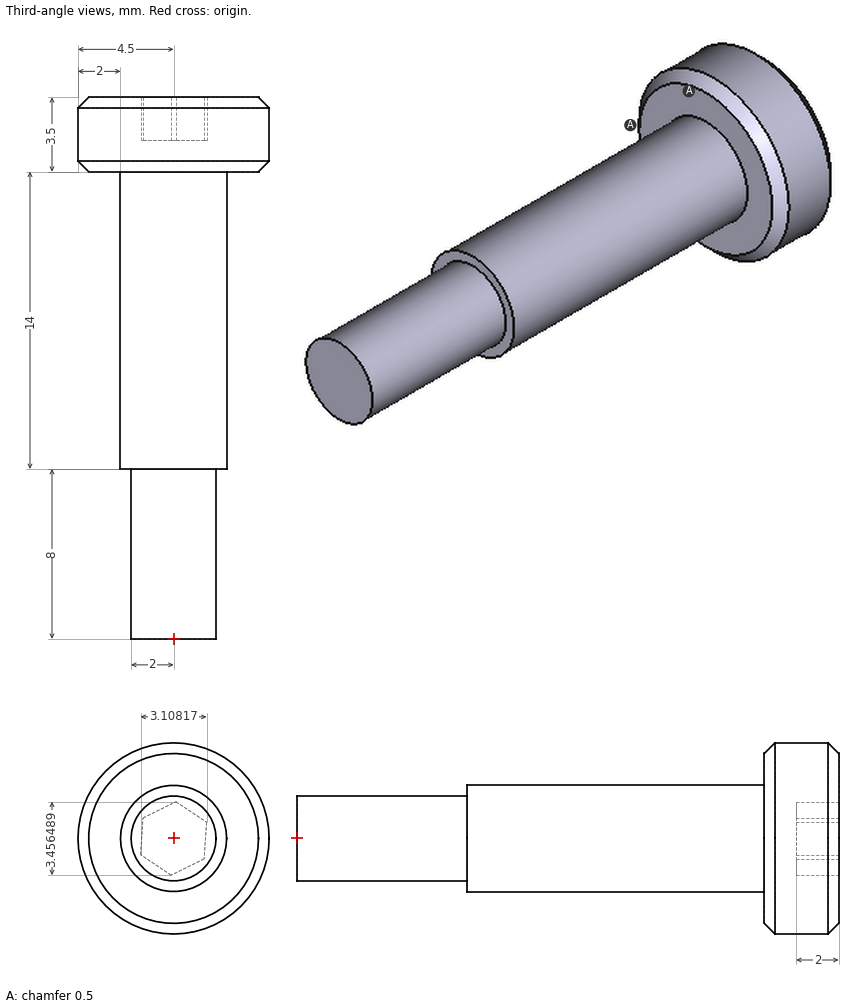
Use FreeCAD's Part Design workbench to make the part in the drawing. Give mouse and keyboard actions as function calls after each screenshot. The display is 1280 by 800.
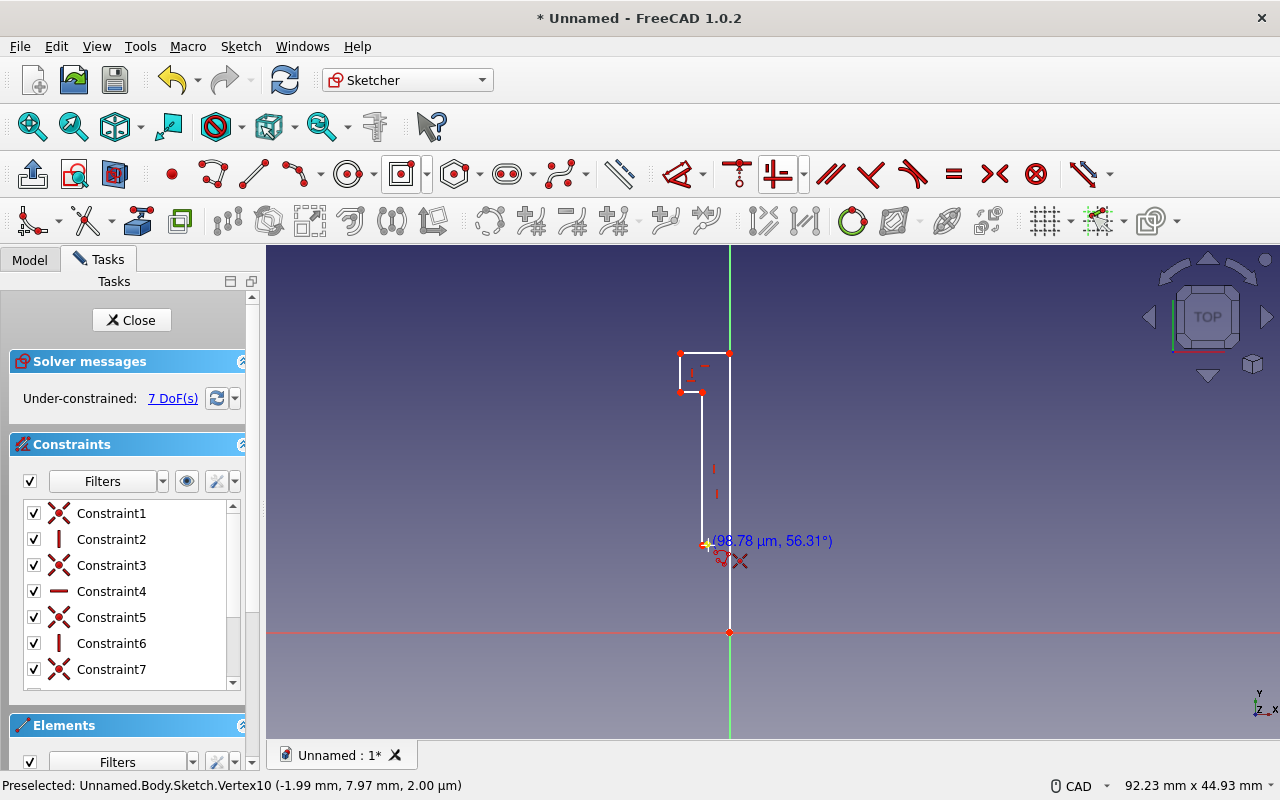
click(708, 624)
click(730, 633)
key(Escape)
key(Escape)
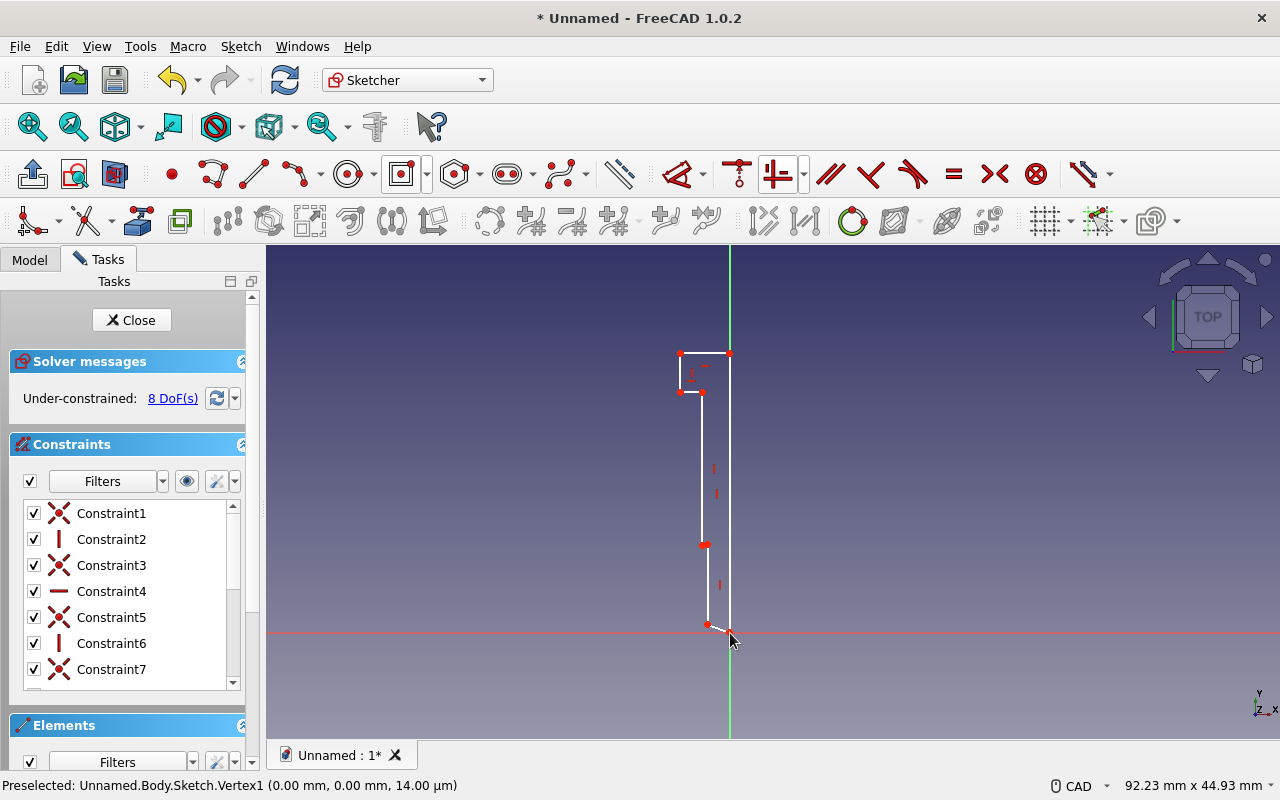
scroll(705, 545, up, 9)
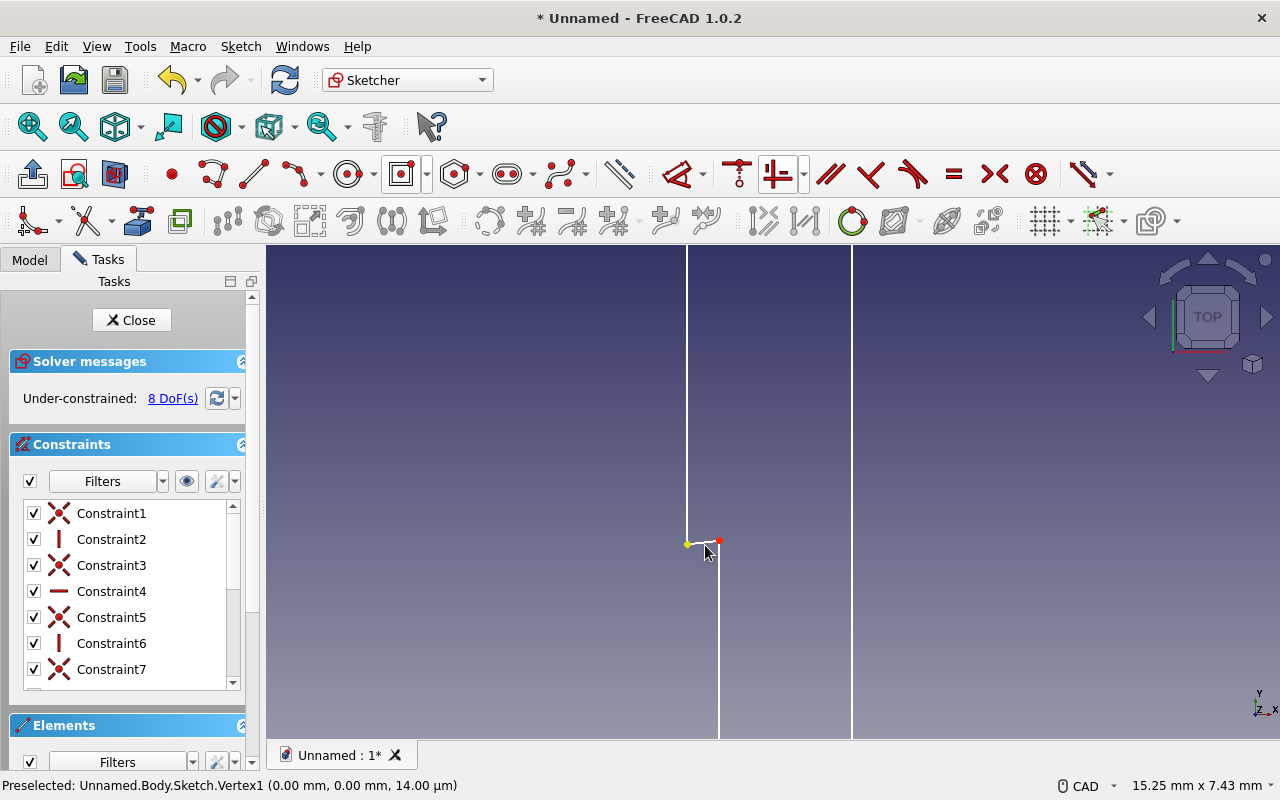
click(703, 543)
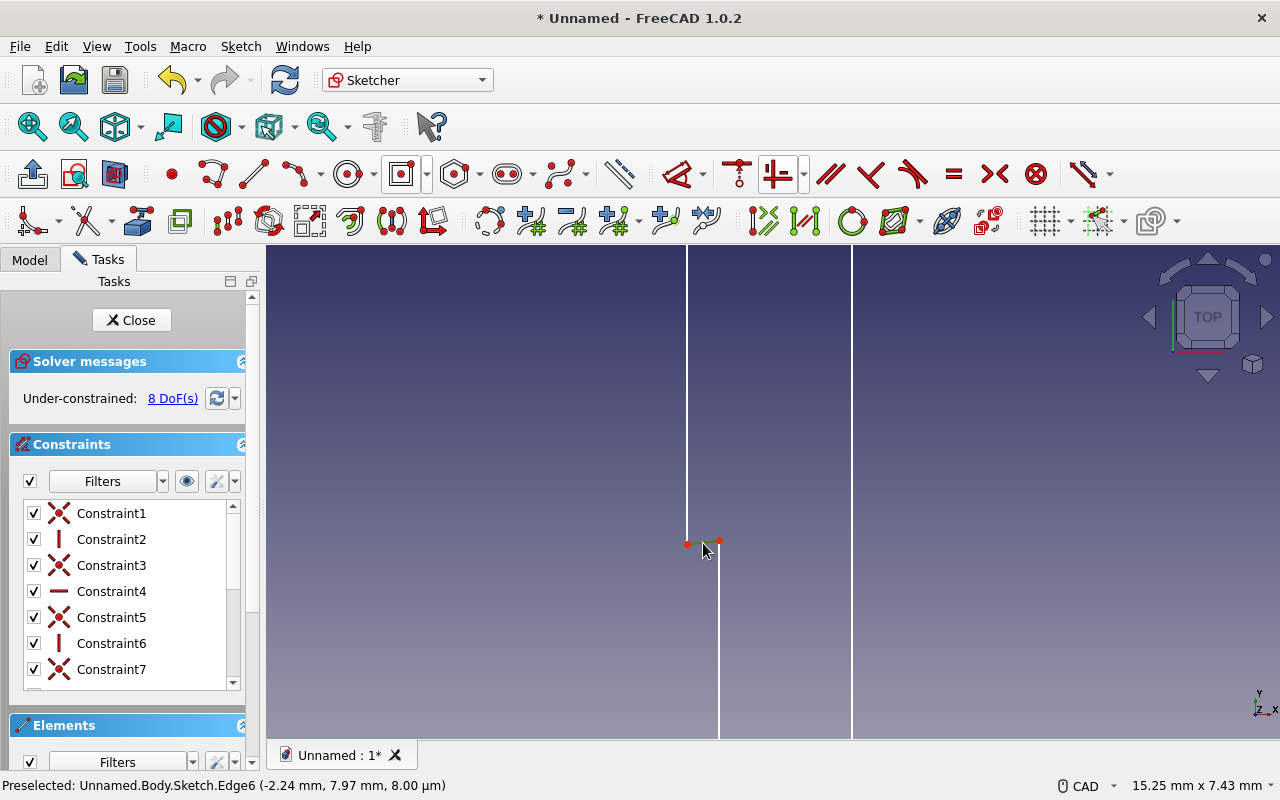
click(804, 174)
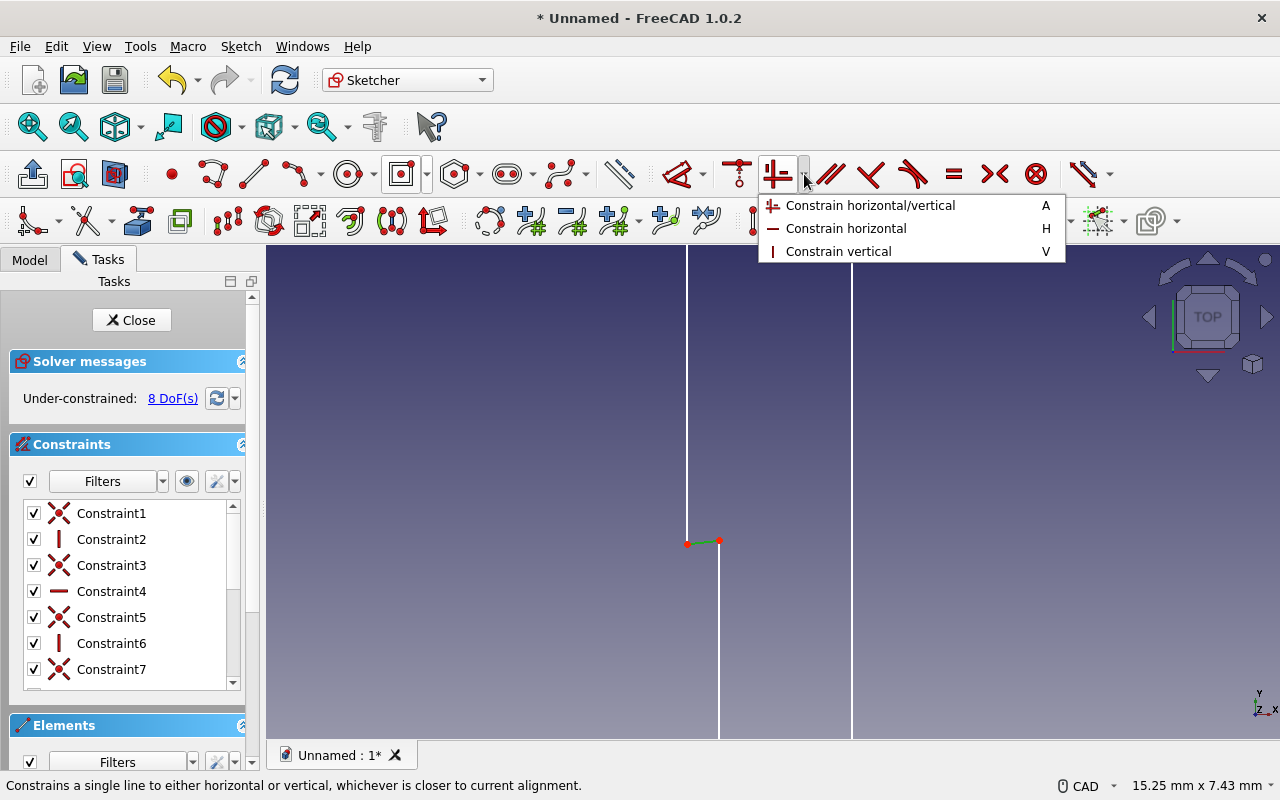
click(912, 228)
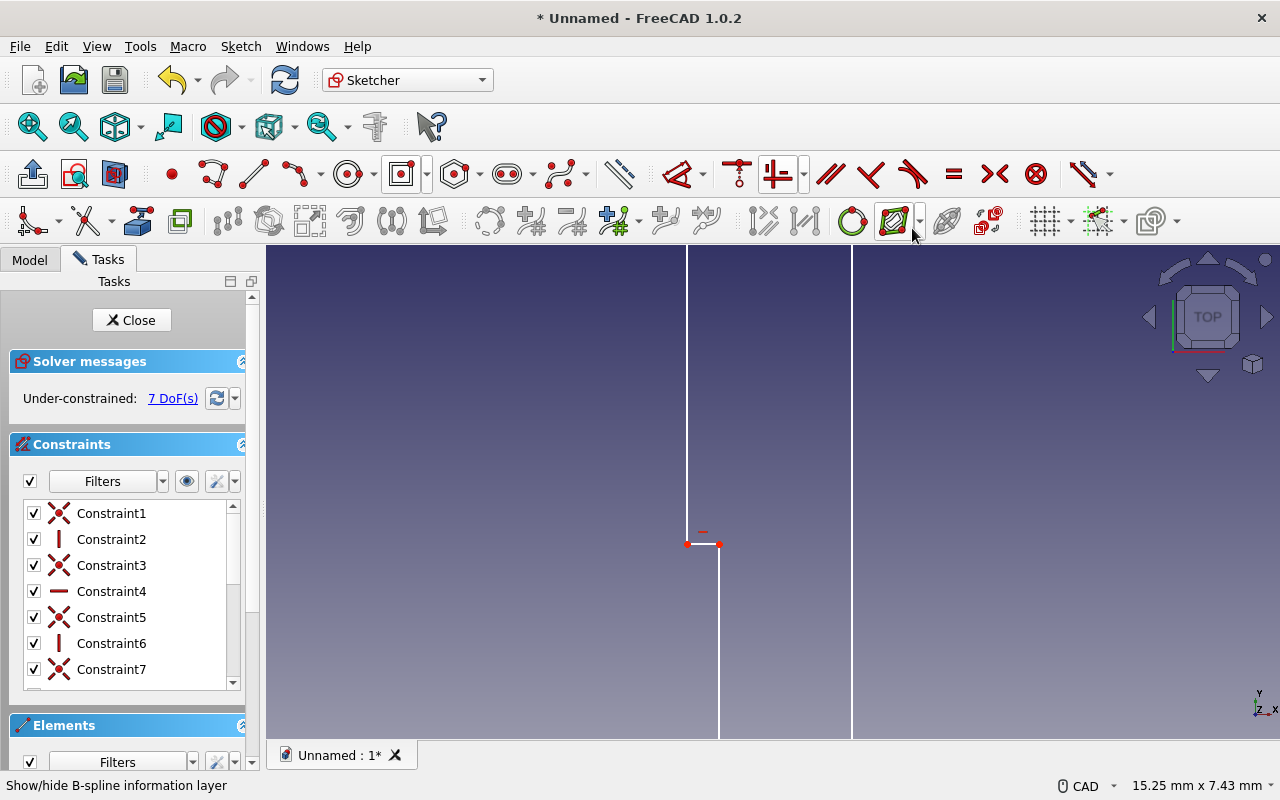
scroll(705, 545, down, 9)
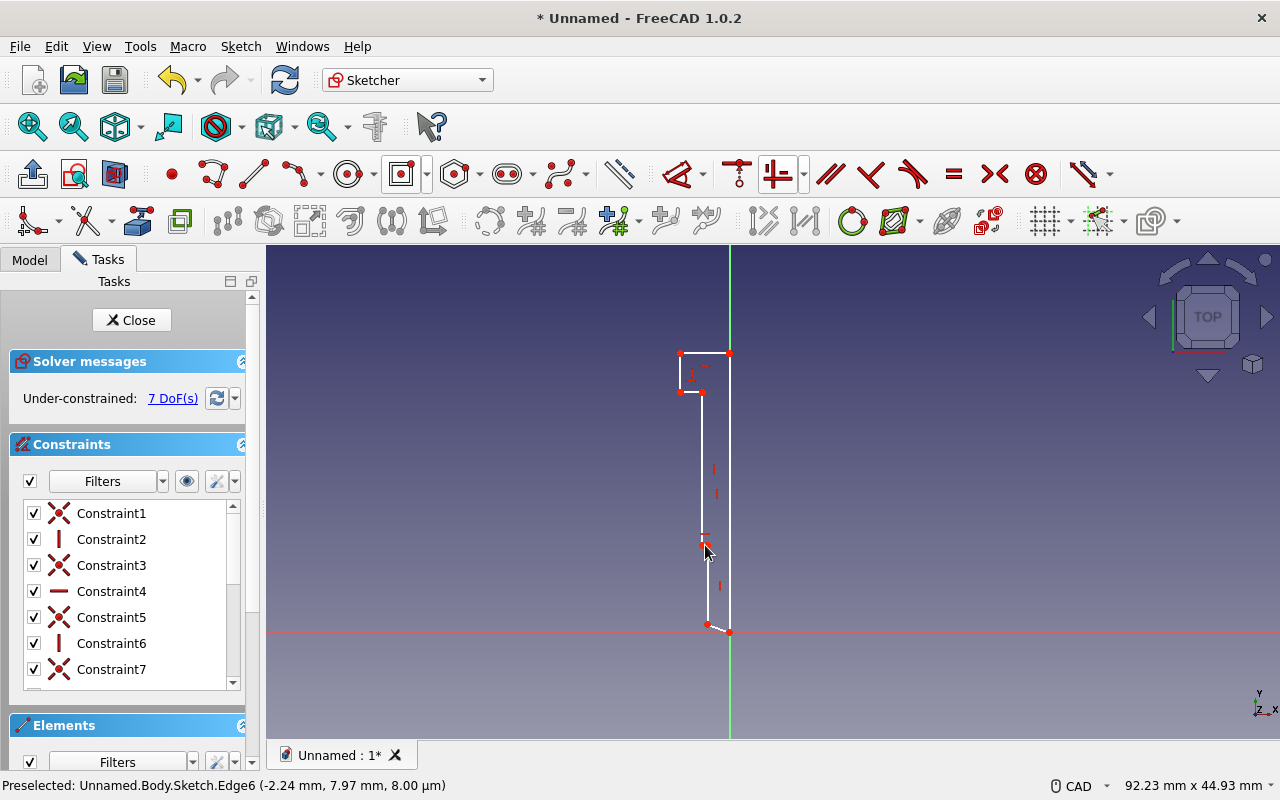
scroll(714, 627, up, 5)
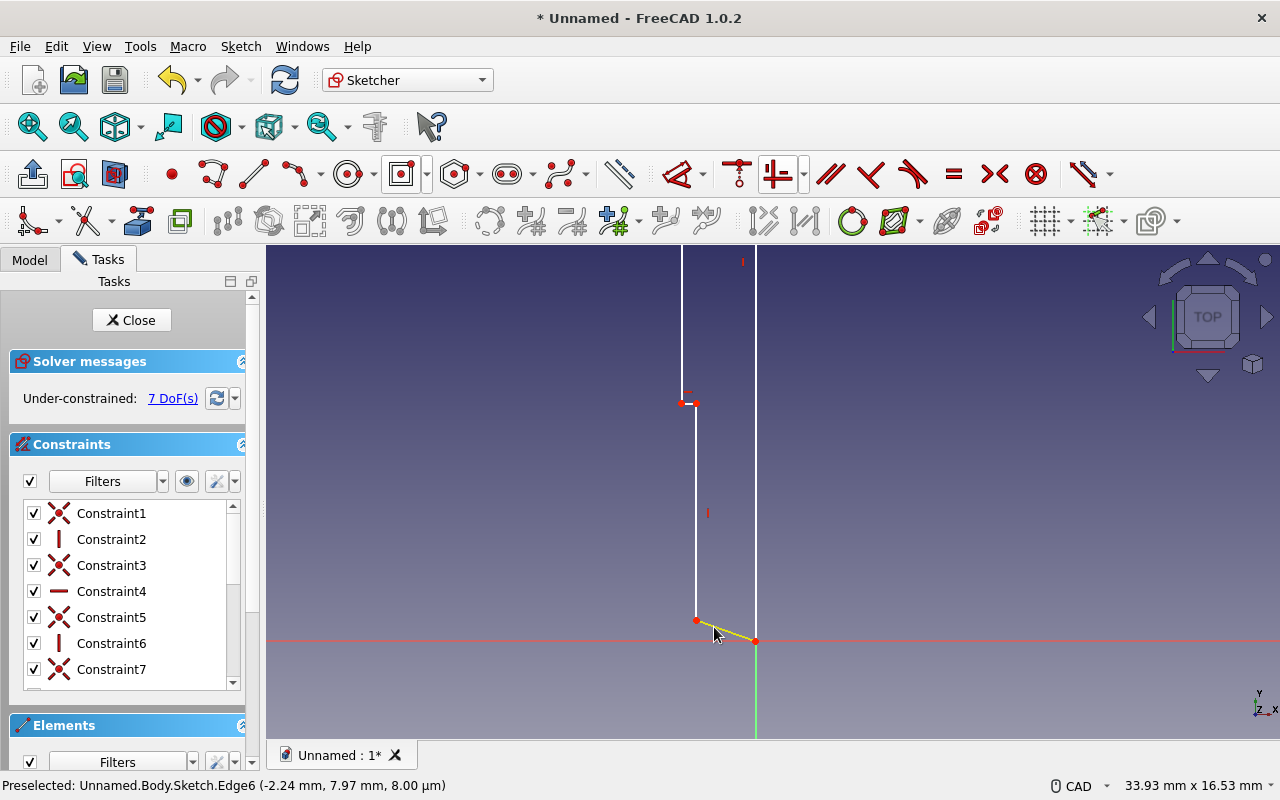
click(714, 627)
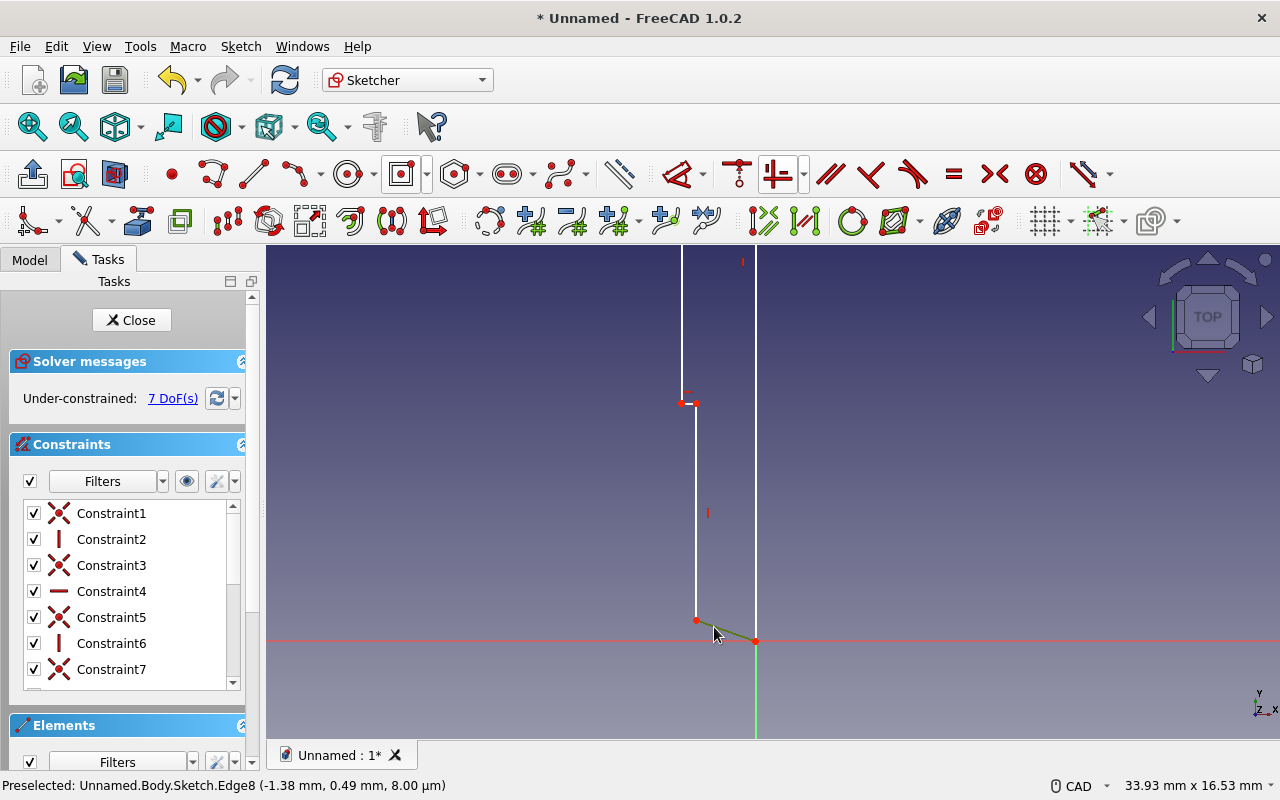
key(h)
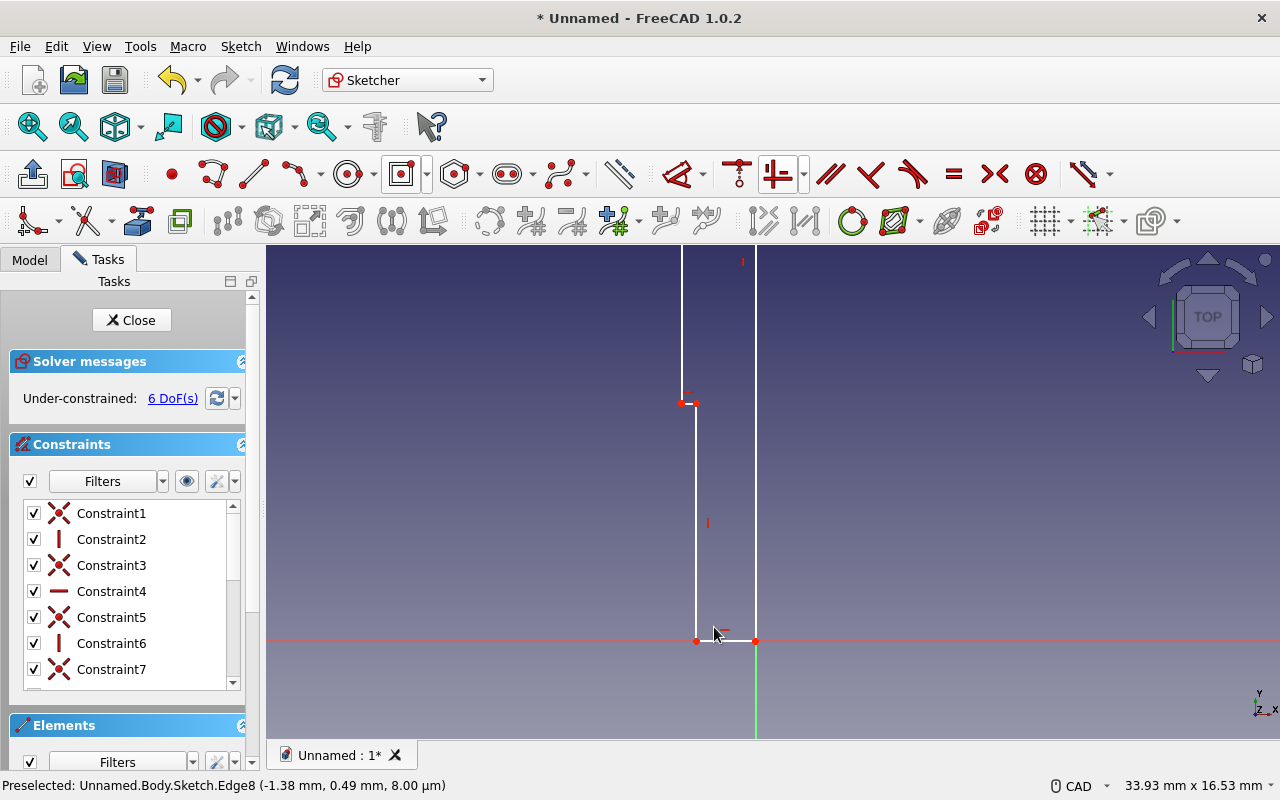
click(676, 174)